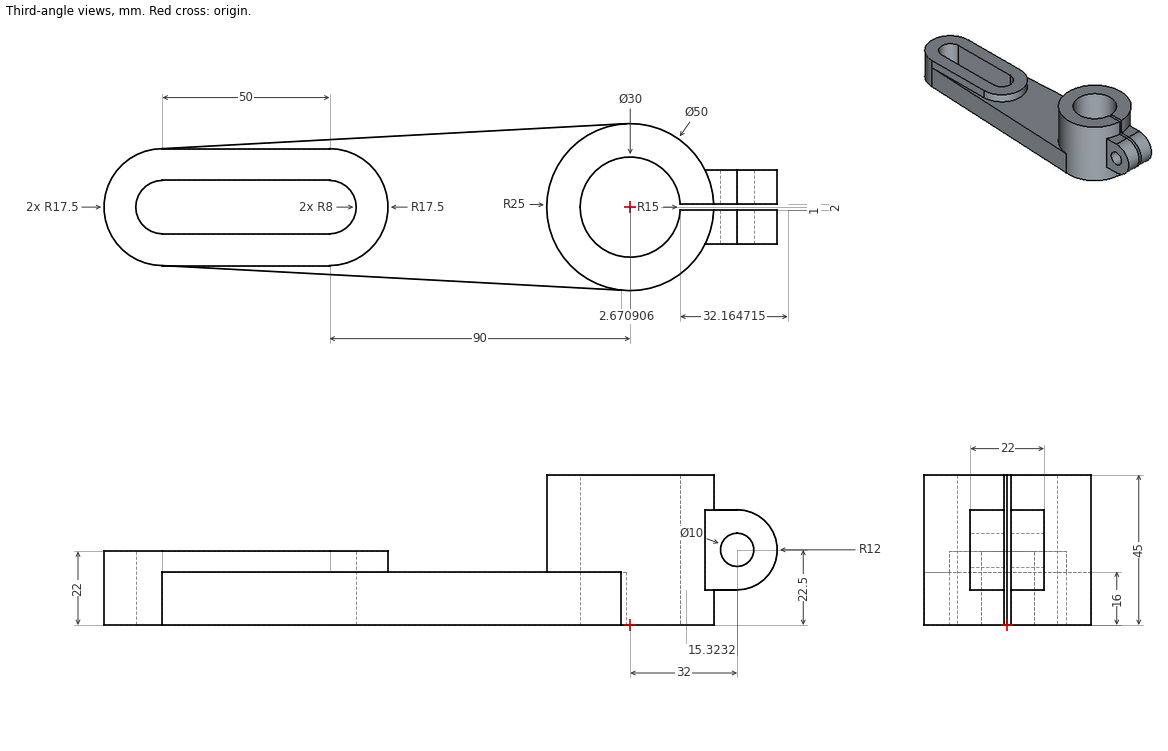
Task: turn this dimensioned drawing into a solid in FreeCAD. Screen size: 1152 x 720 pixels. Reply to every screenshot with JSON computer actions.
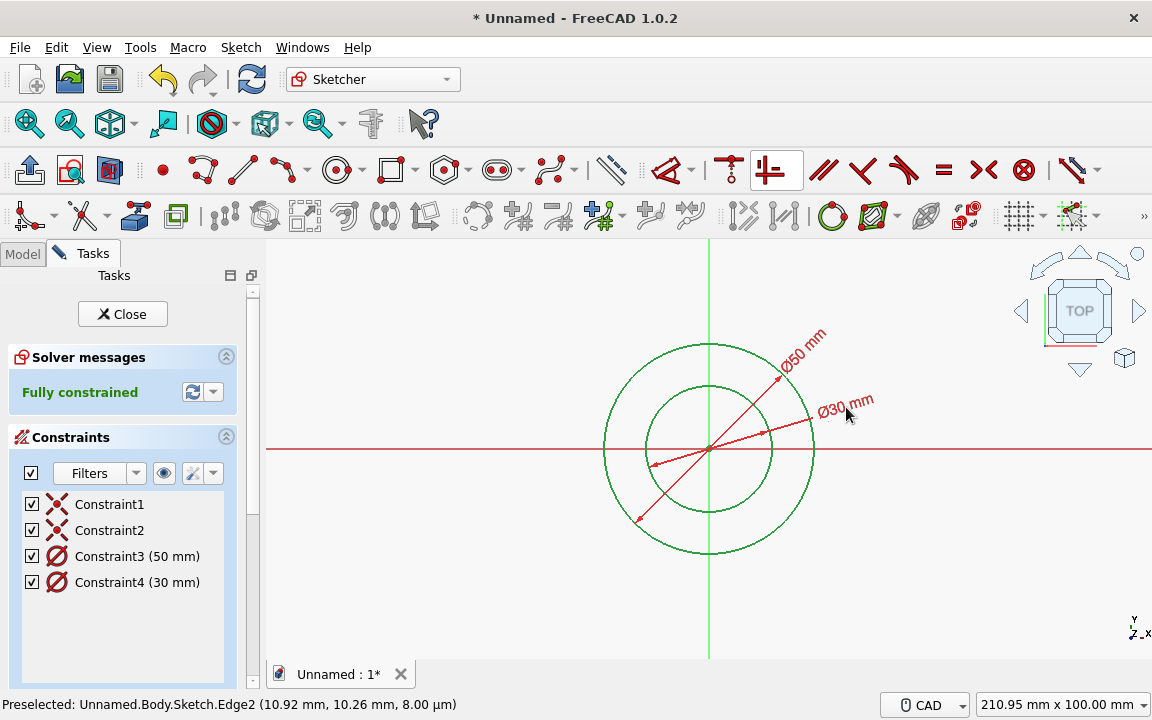
{"action": "left_click", "coordinate": [123, 314]}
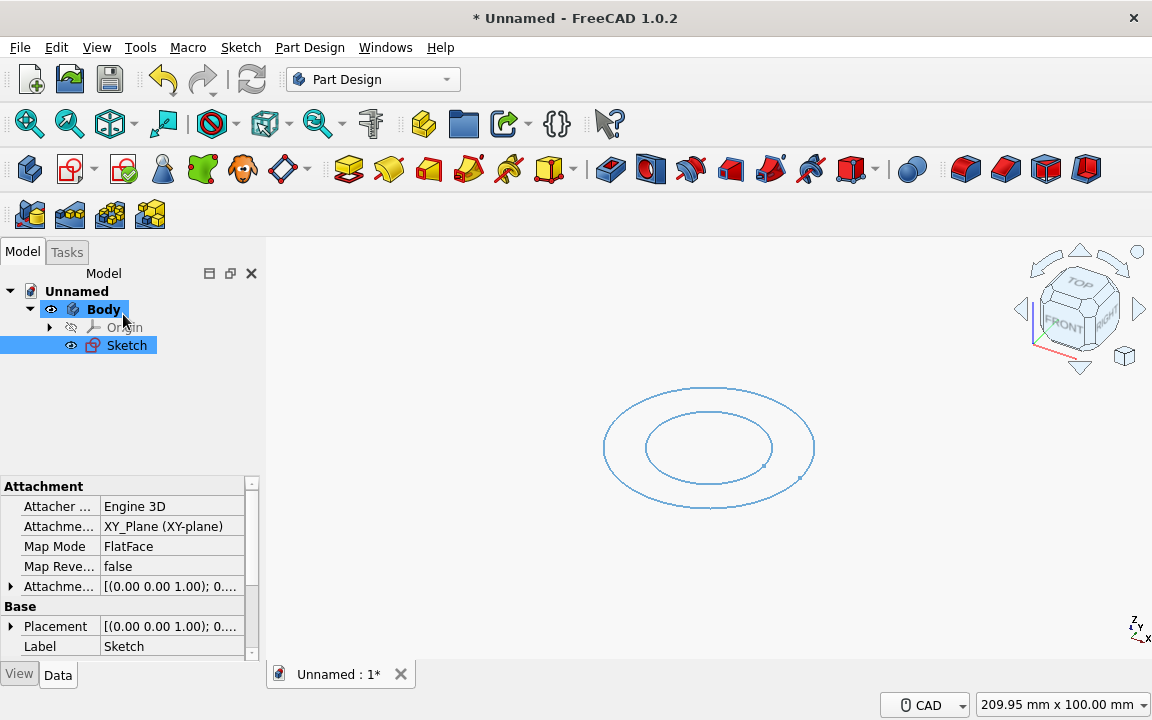
{"action": "left_click", "coordinate": [350, 170]}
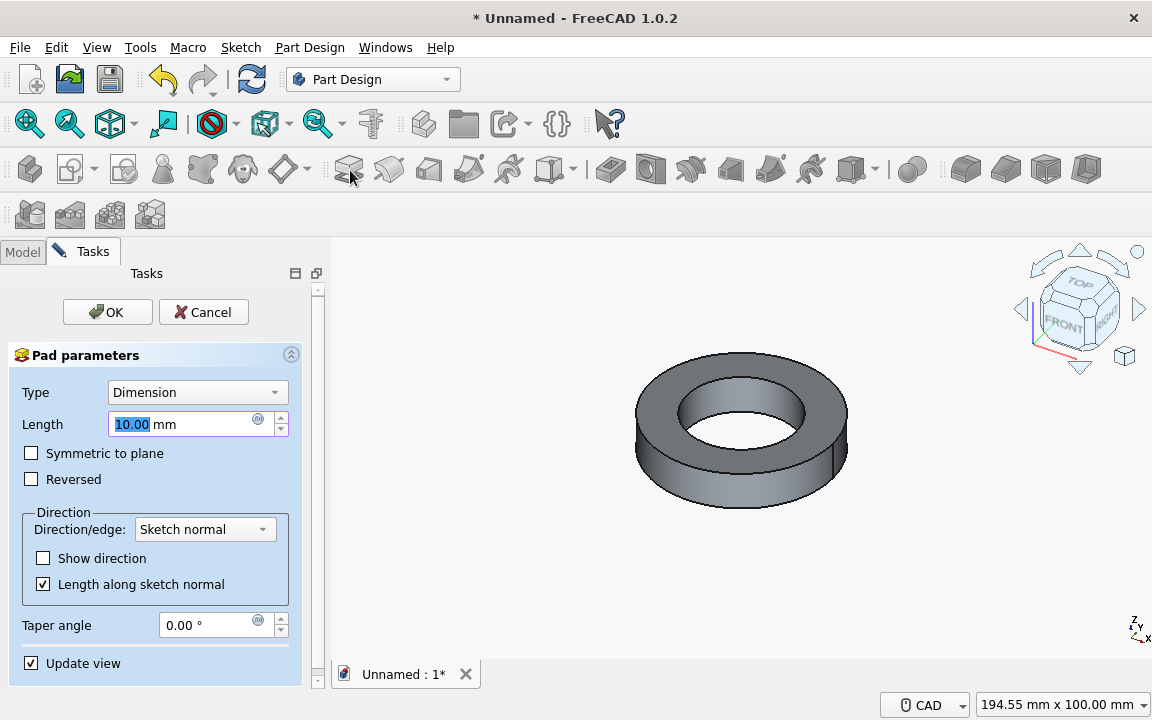
{"action": "type", "text": "45"}
{"action": "key", "text": "Tab"}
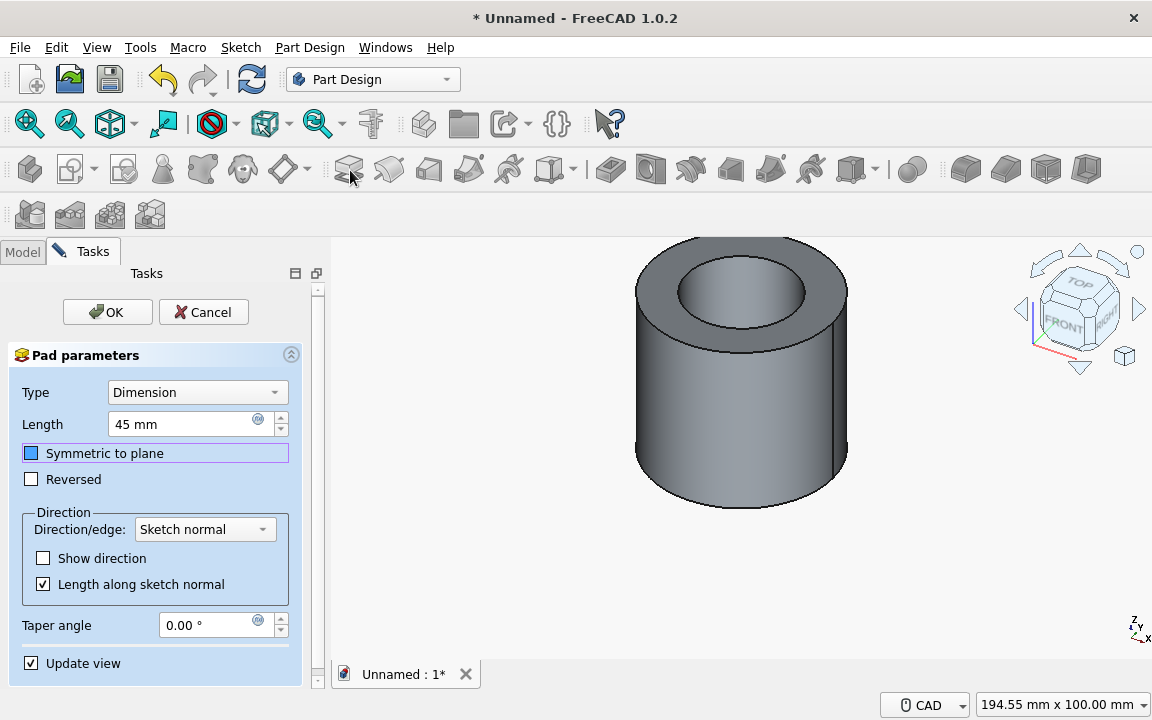
{"action": "left_click", "coordinate": [108, 312]}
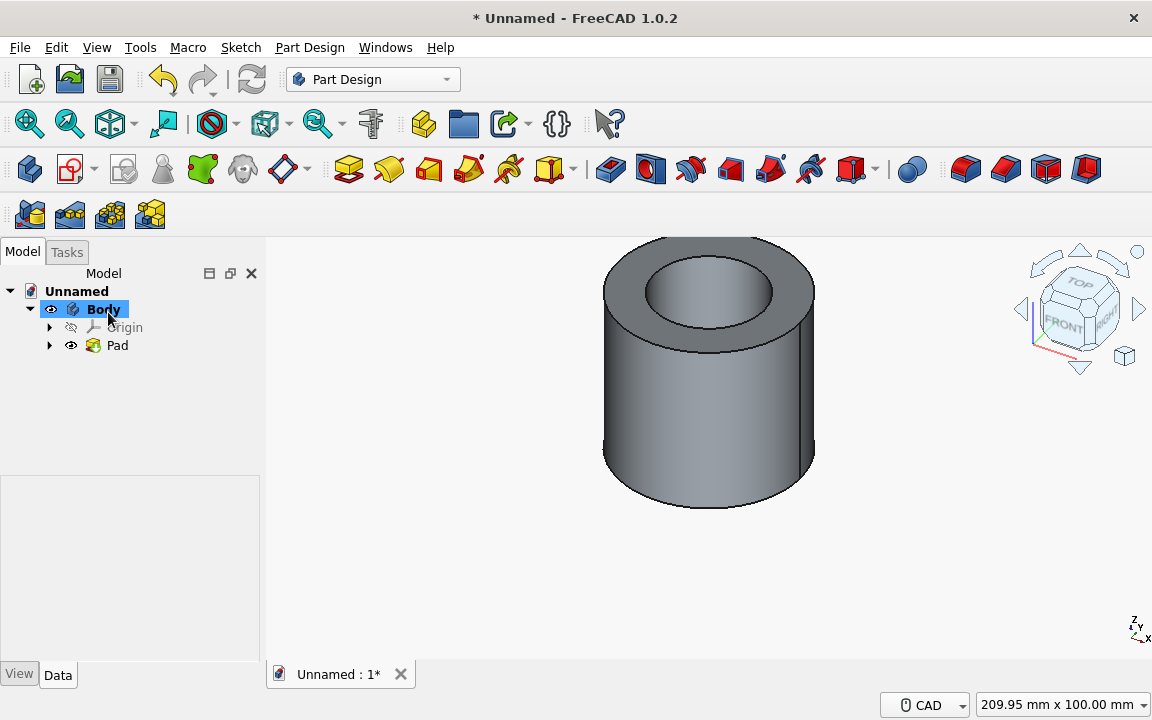
{"action": "key", "text": "v f"}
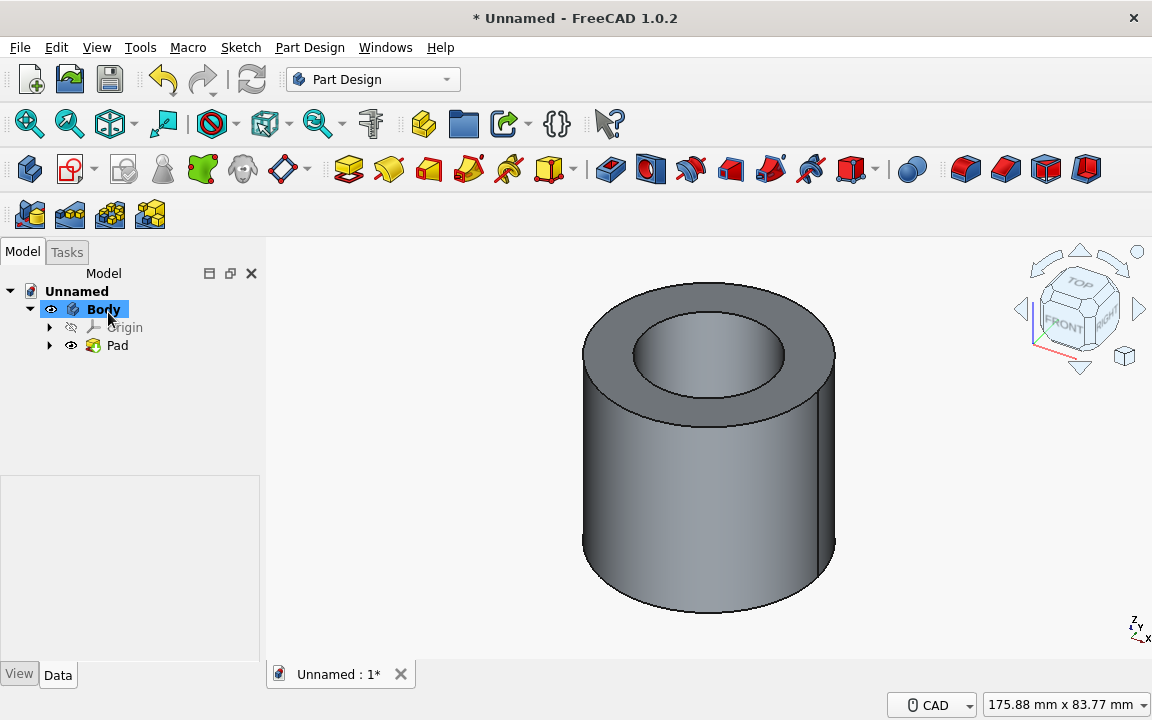
{"action": "left_click", "coordinate": [30, 170]}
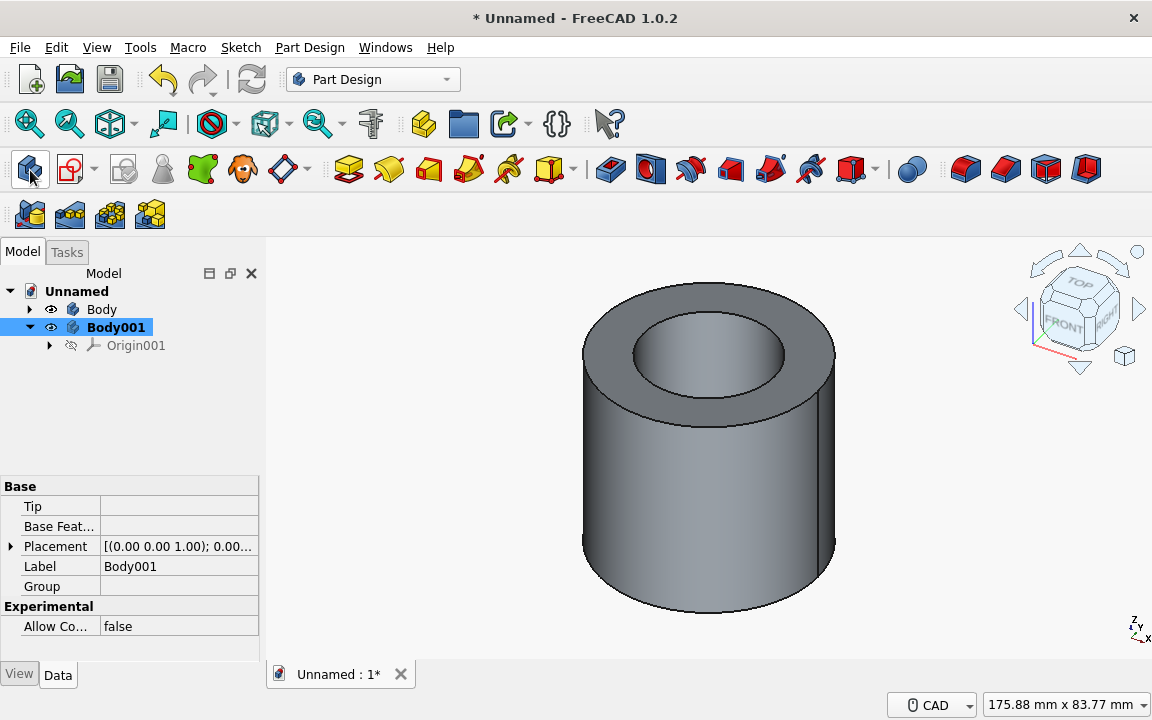
{"action": "left_click", "coordinate": [306, 619]}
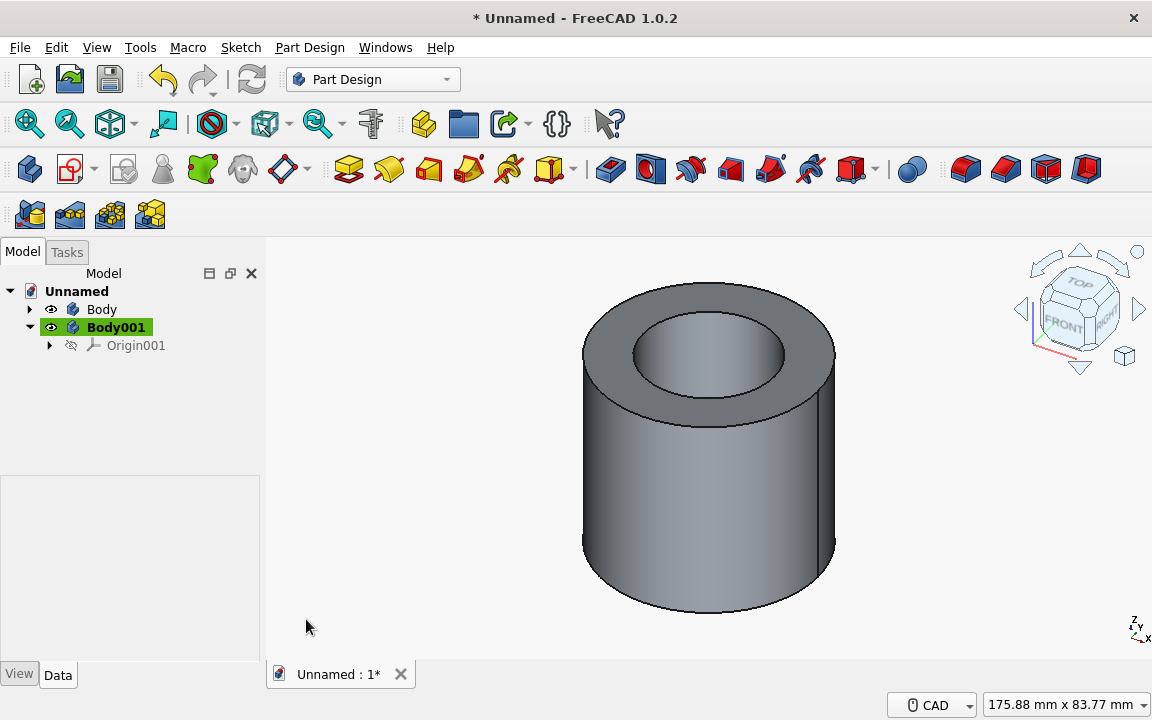
{"action": "left_click", "coordinate": [70, 170]}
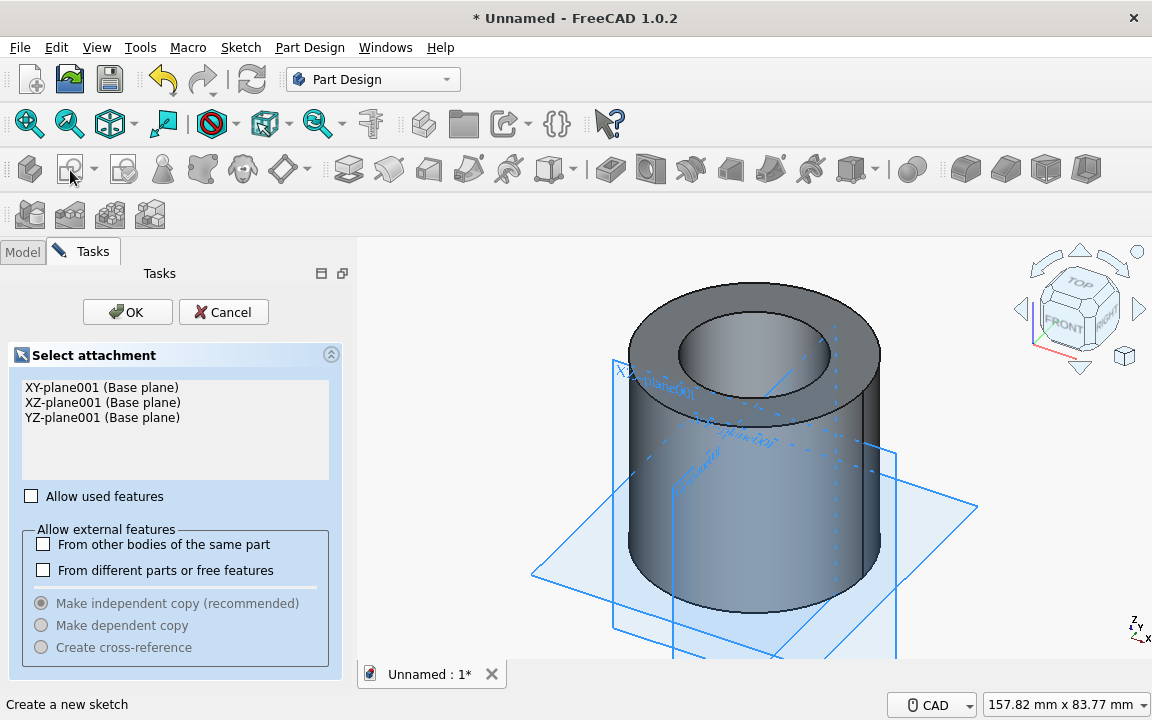
{"action": "left_click", "coordinate": [82, 388]}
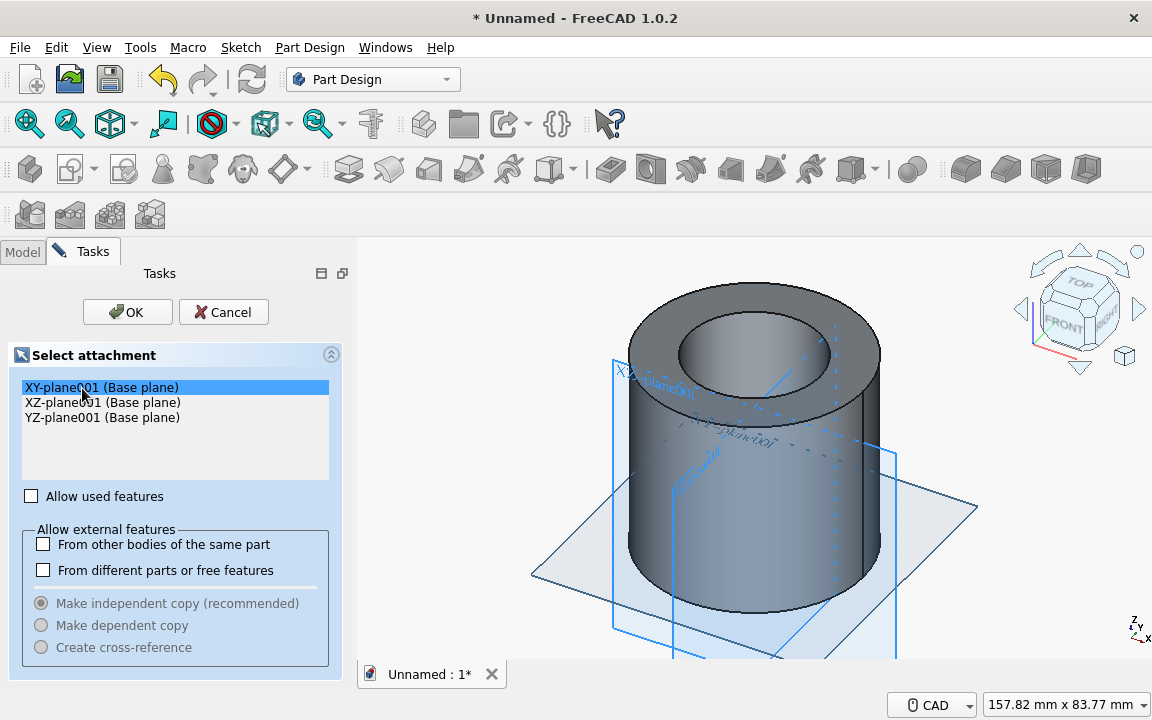
{"action": "left_click", "coordinate": [128, 312]}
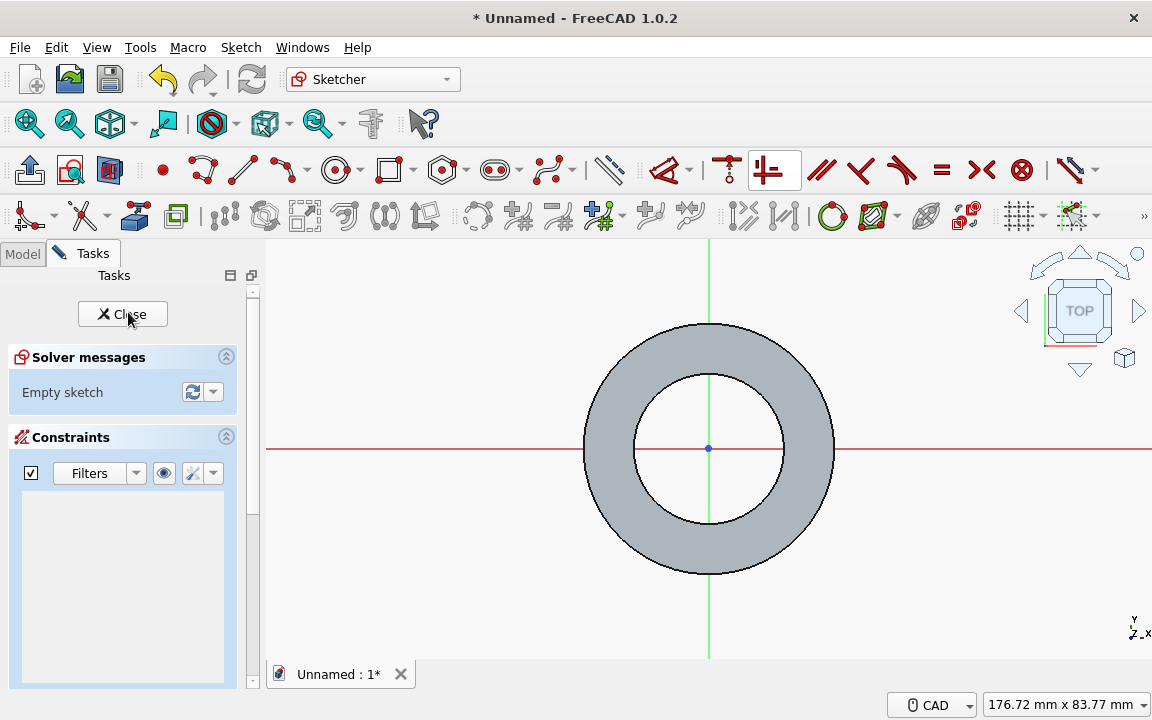
{"action": "scroll", "coordinate": [987, 449], "scroll_direction": "down", "scroll_amount": 3}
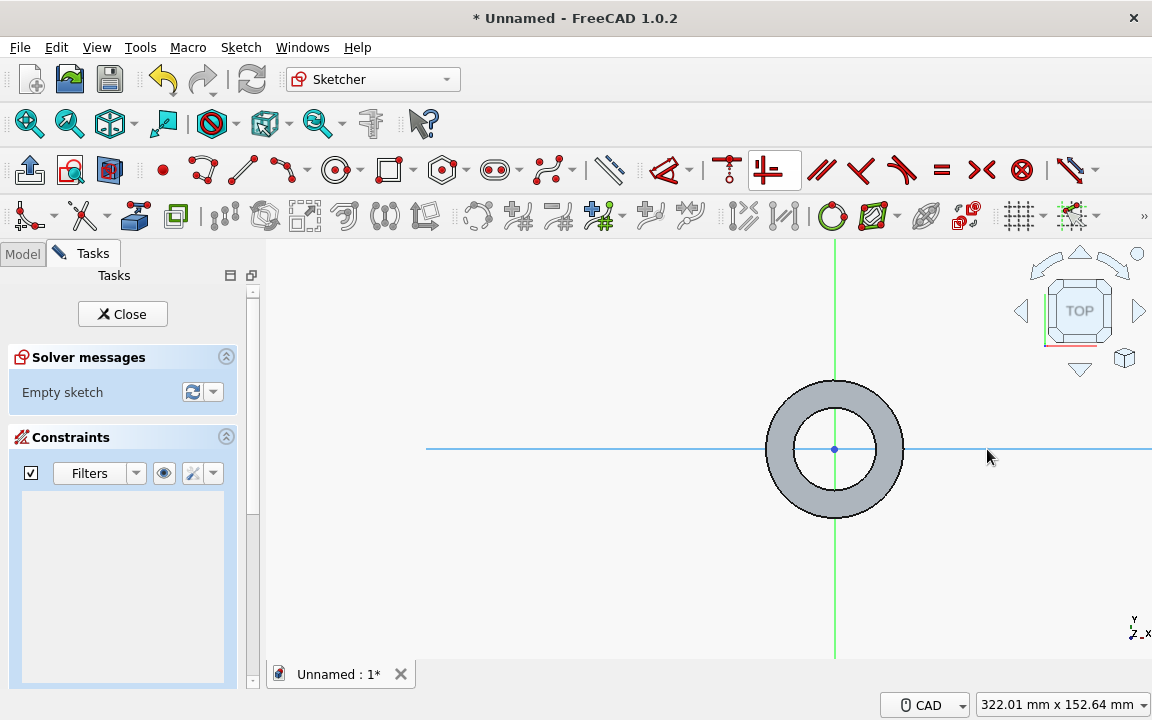
{"action": "left_click", "coordinate": [496, 170]}